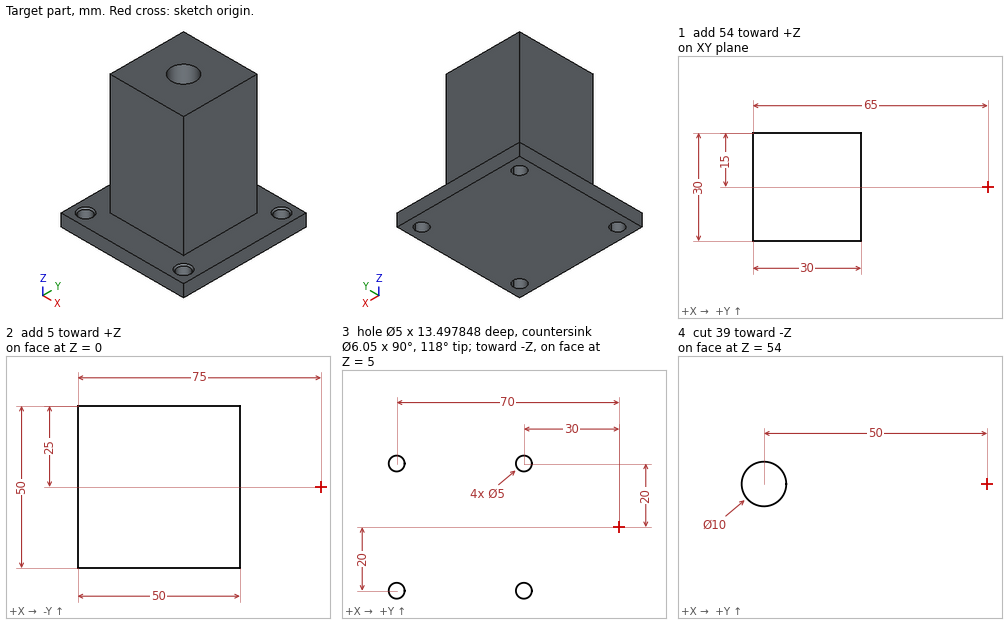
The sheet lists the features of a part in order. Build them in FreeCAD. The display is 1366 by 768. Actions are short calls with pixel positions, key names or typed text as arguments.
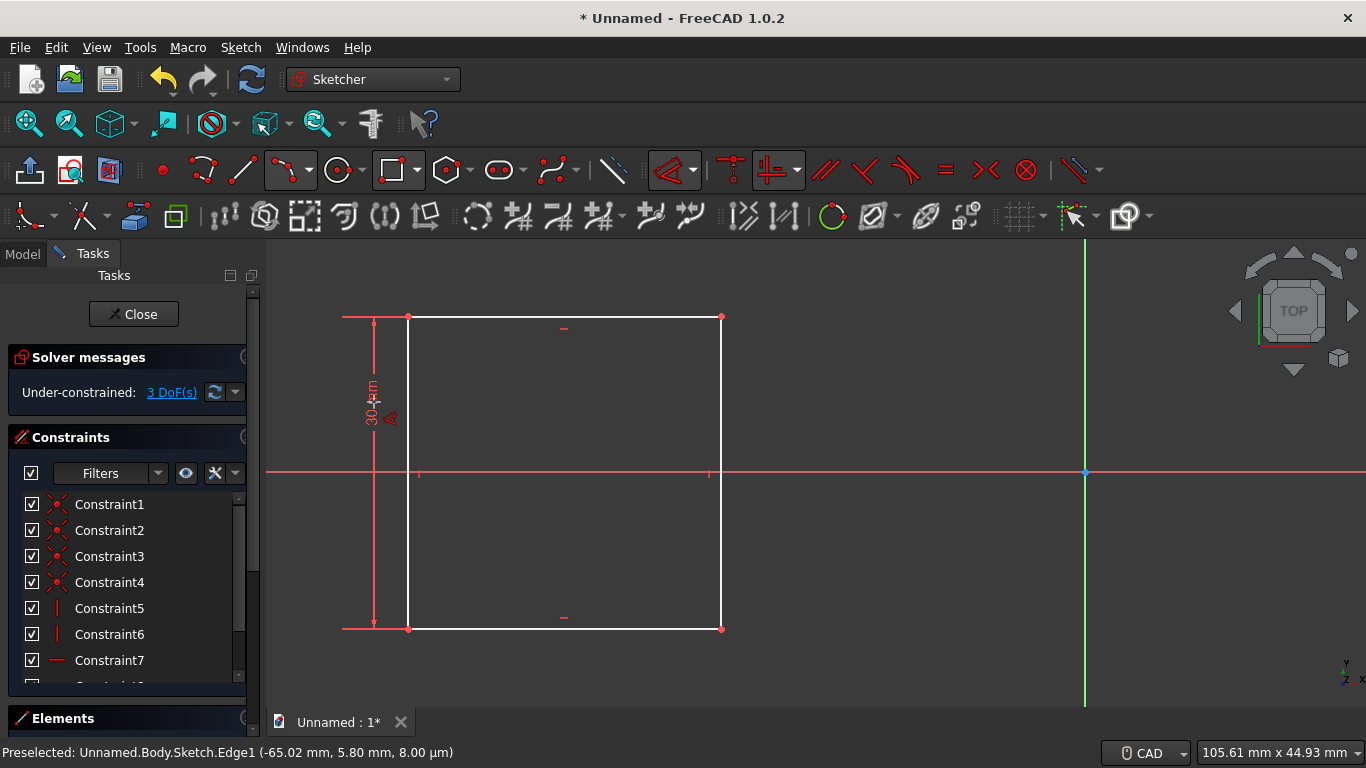
click(502, 629)
click(564, 663)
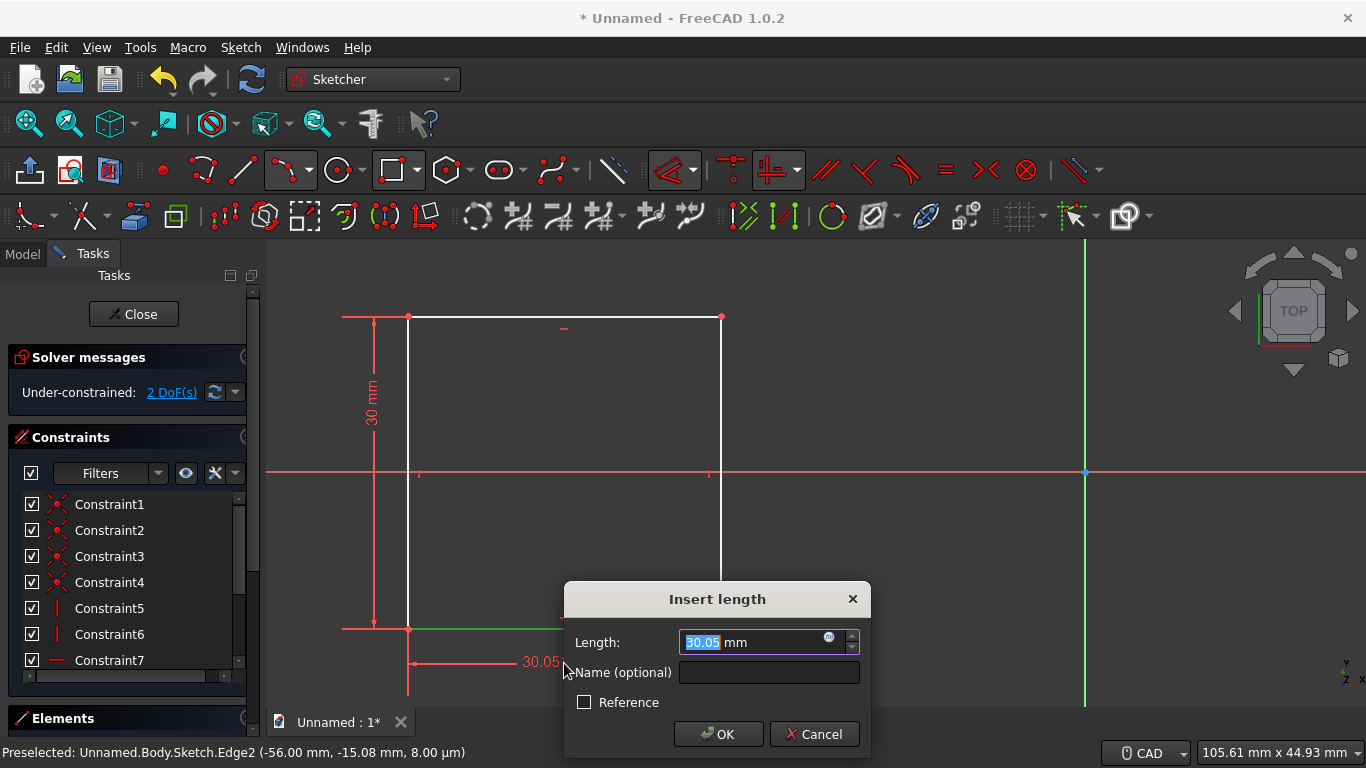
text(30)
key(Return)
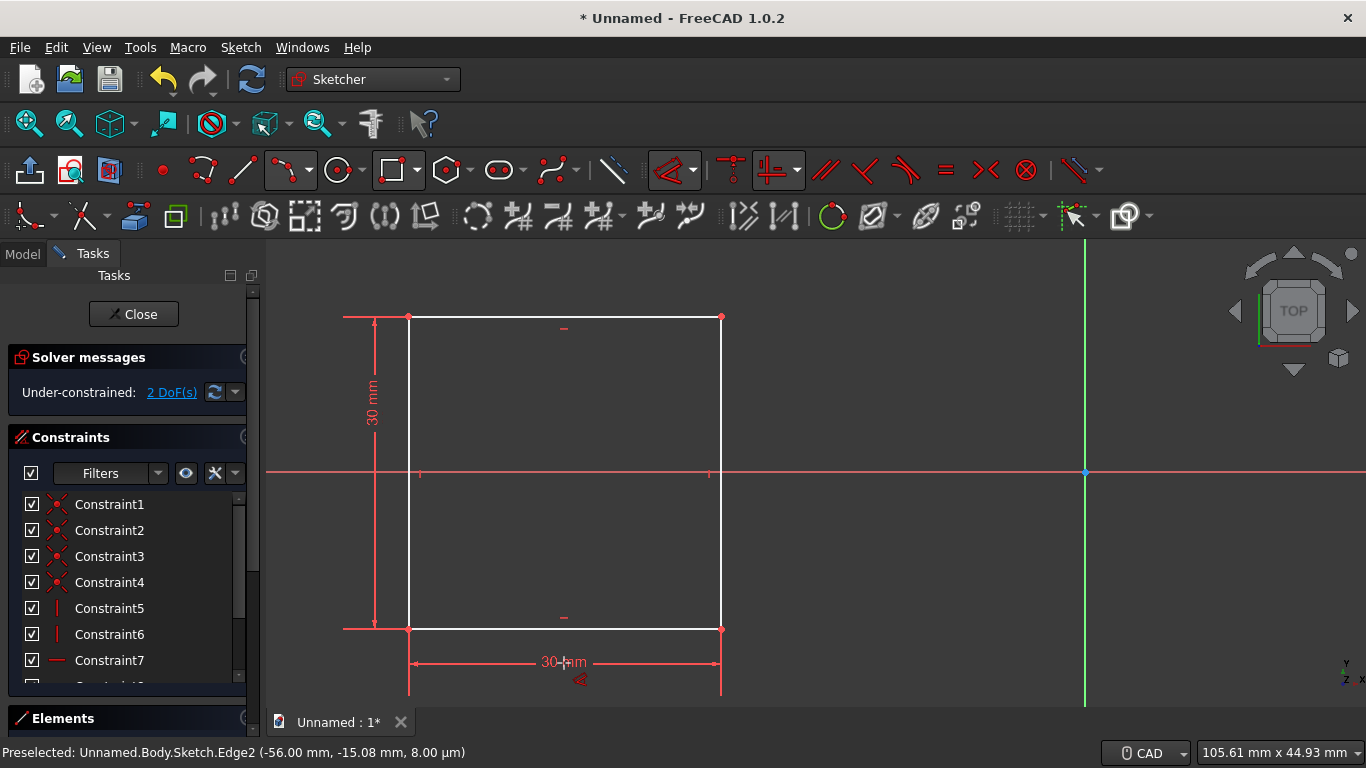
click(409, 317)
click(747, 283)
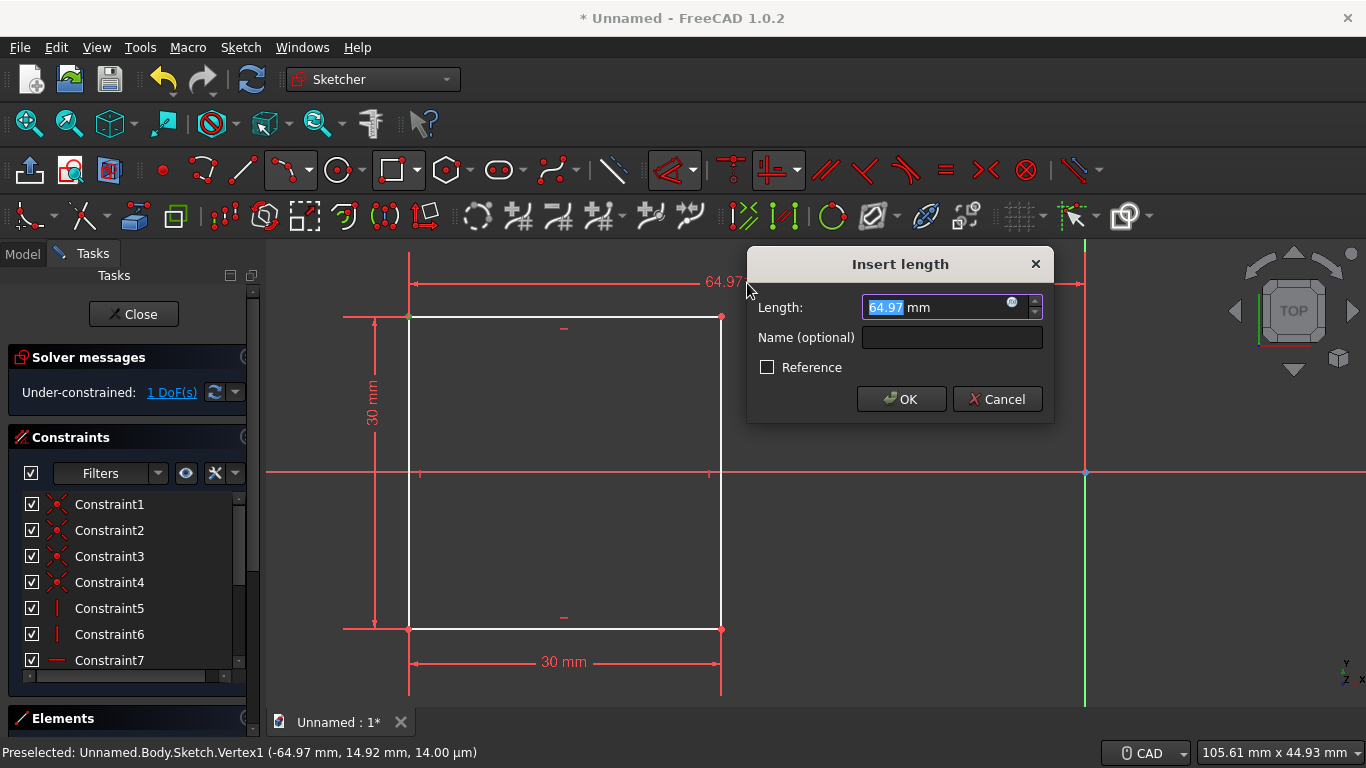
text(65)
key(Return)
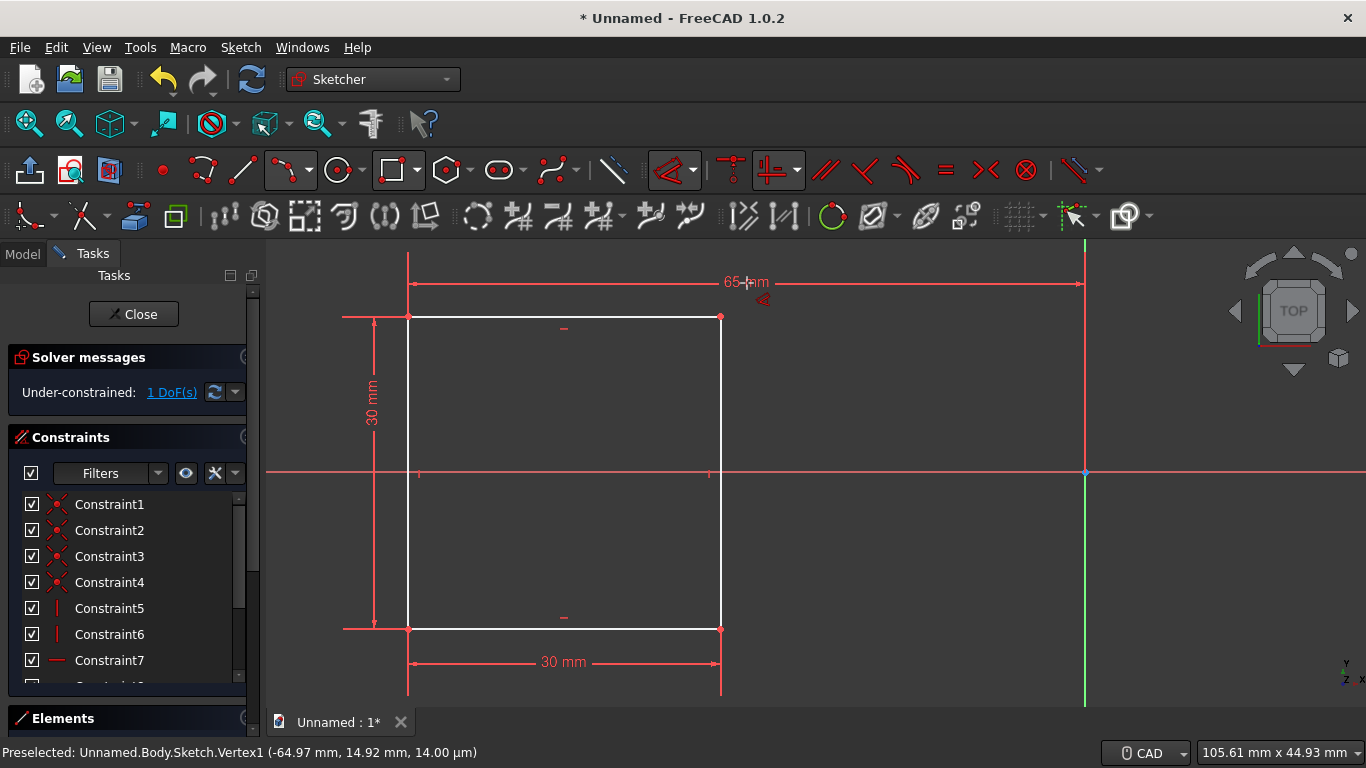
click(408, 317)
click(1119, 395)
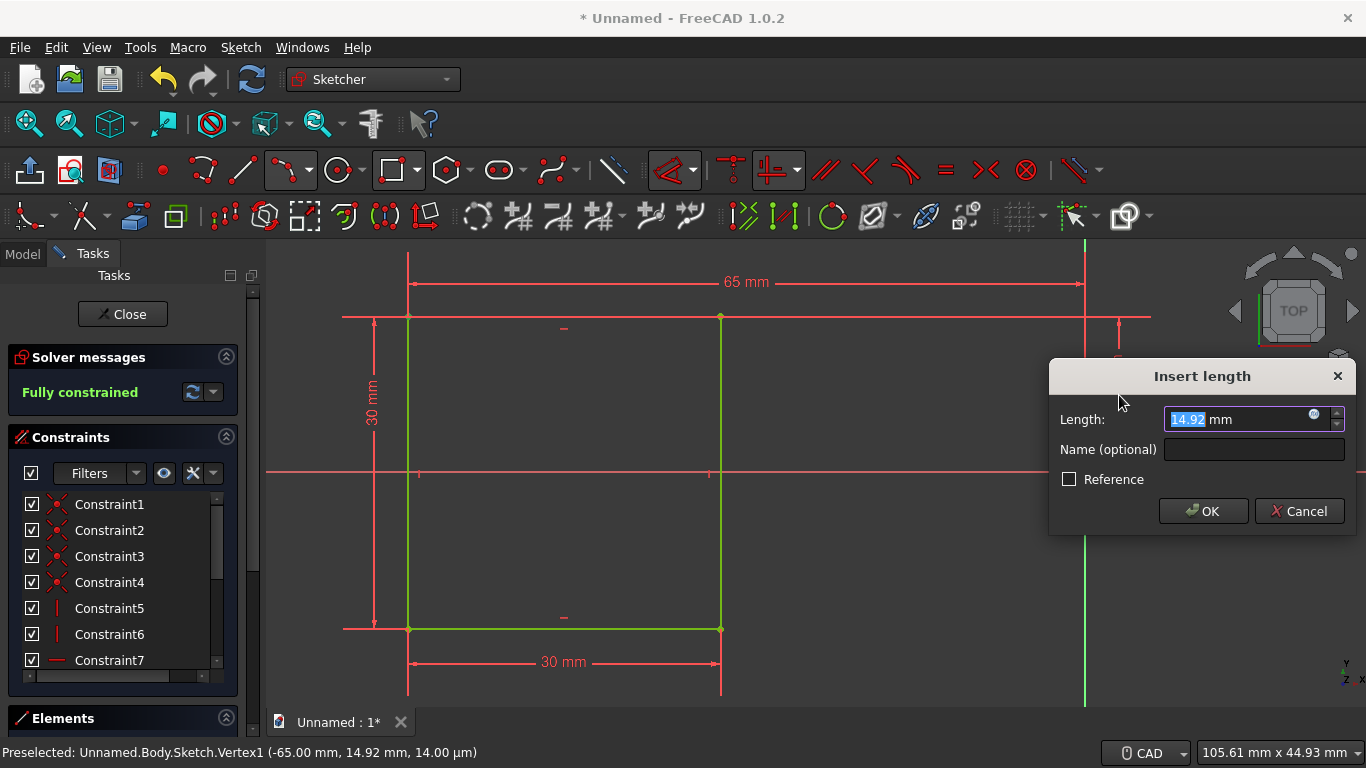
text(15)
key(Return)
key(Escape)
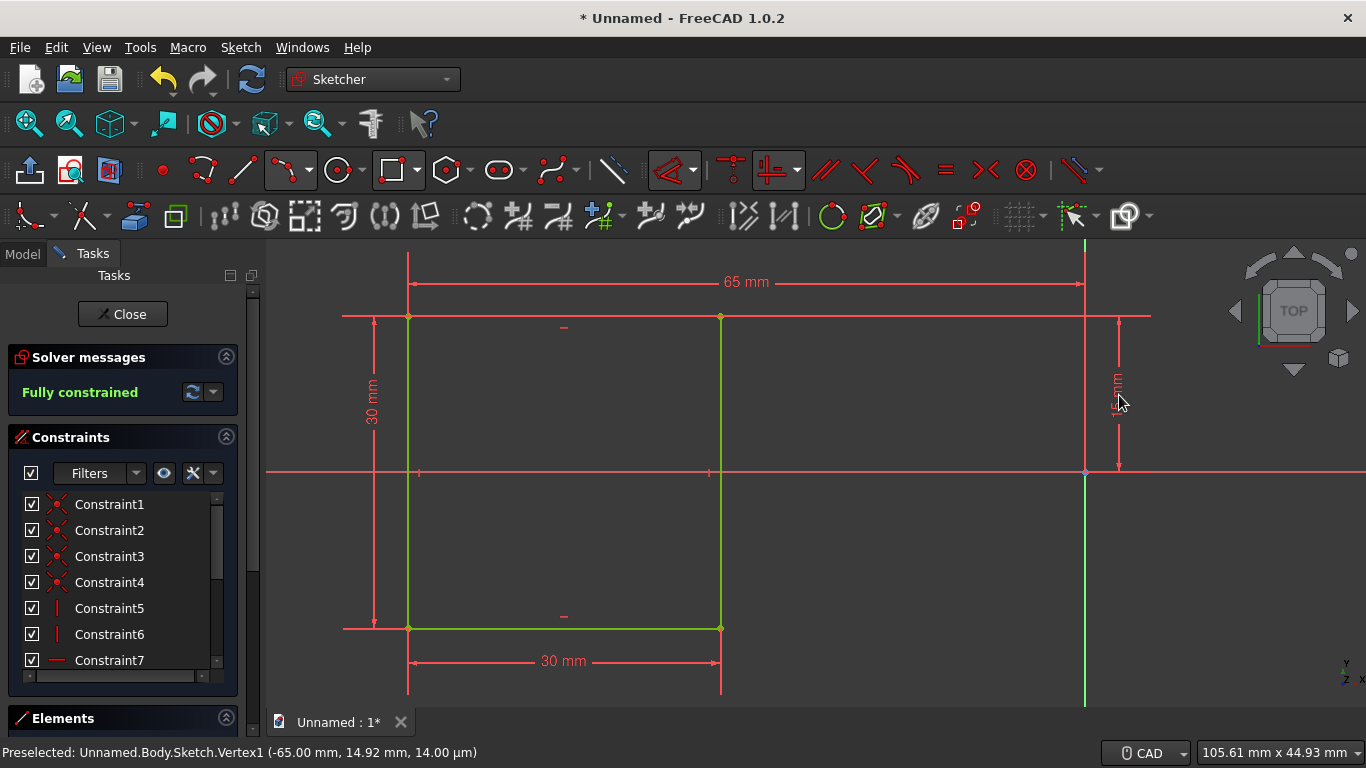
click(123, 314)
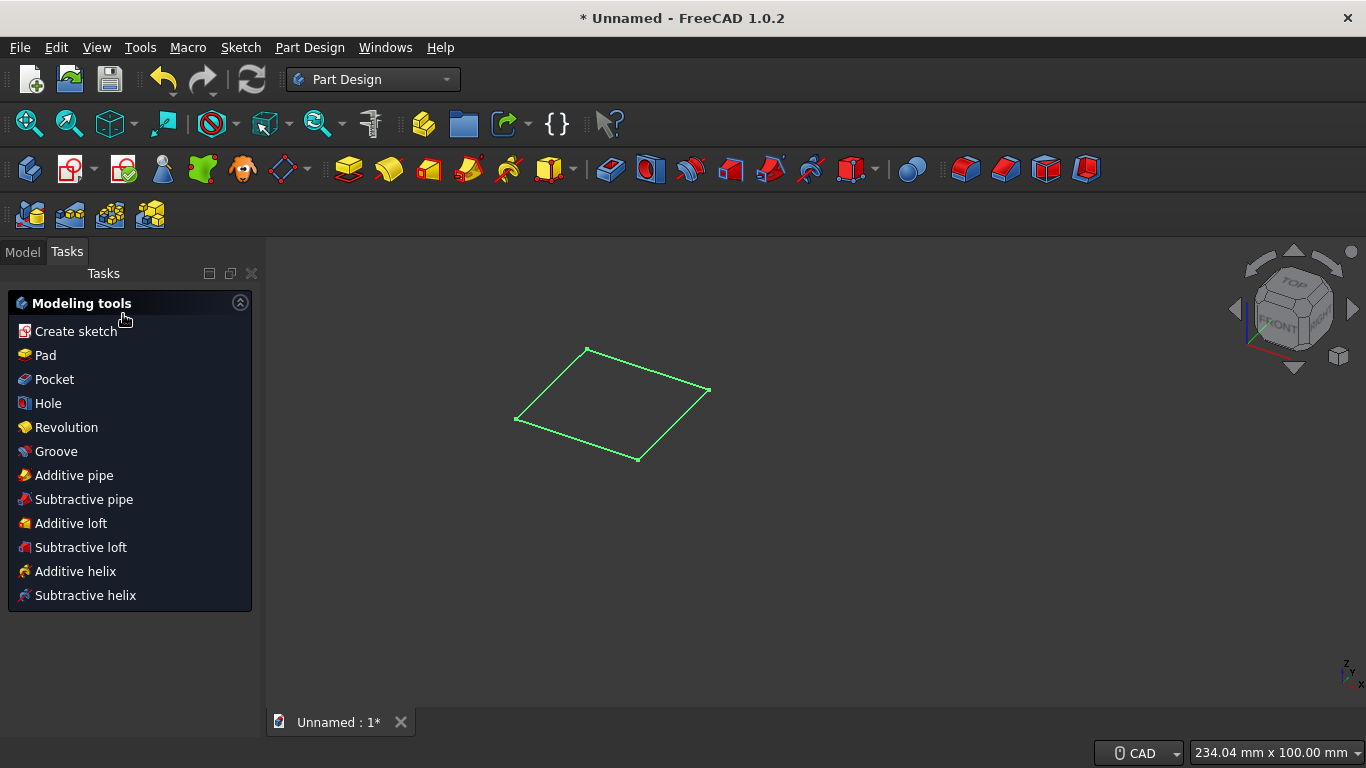
click(350, 170)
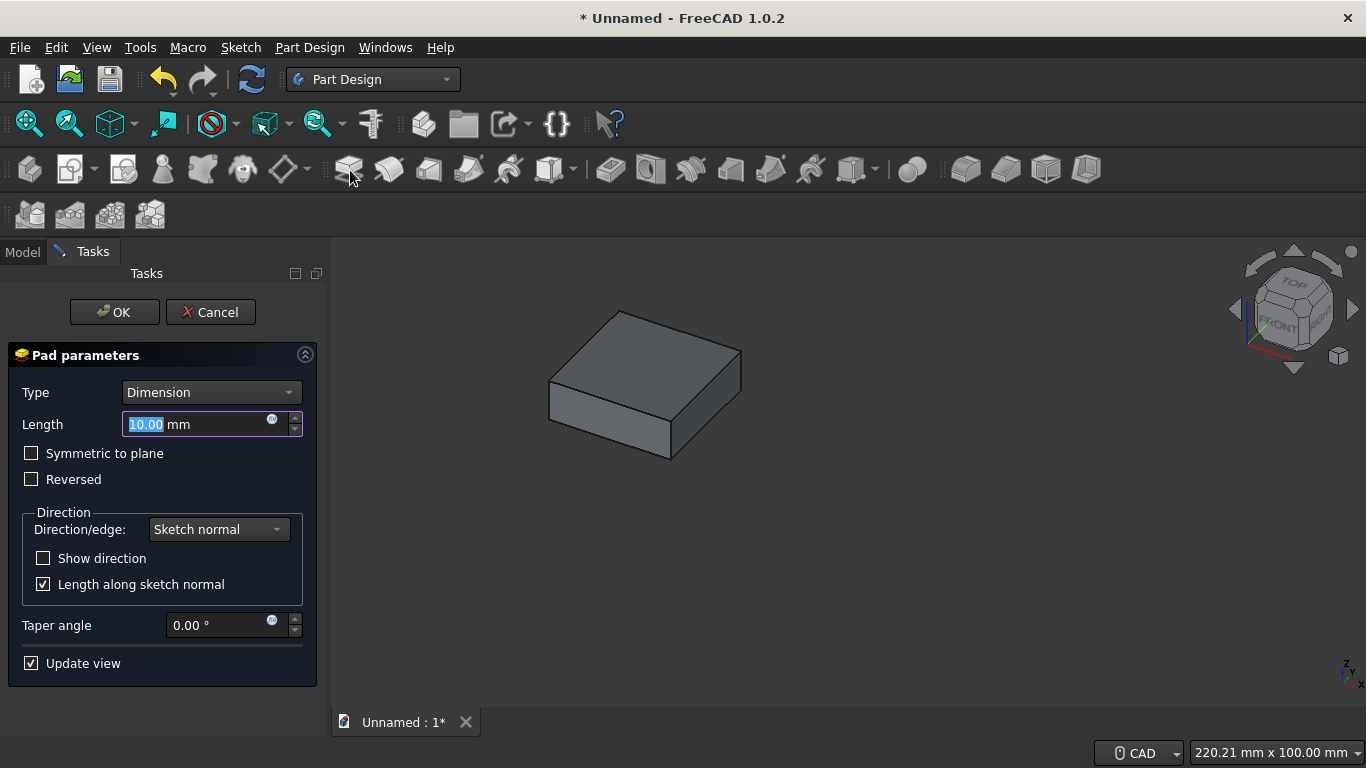
text(54)
key(Tab)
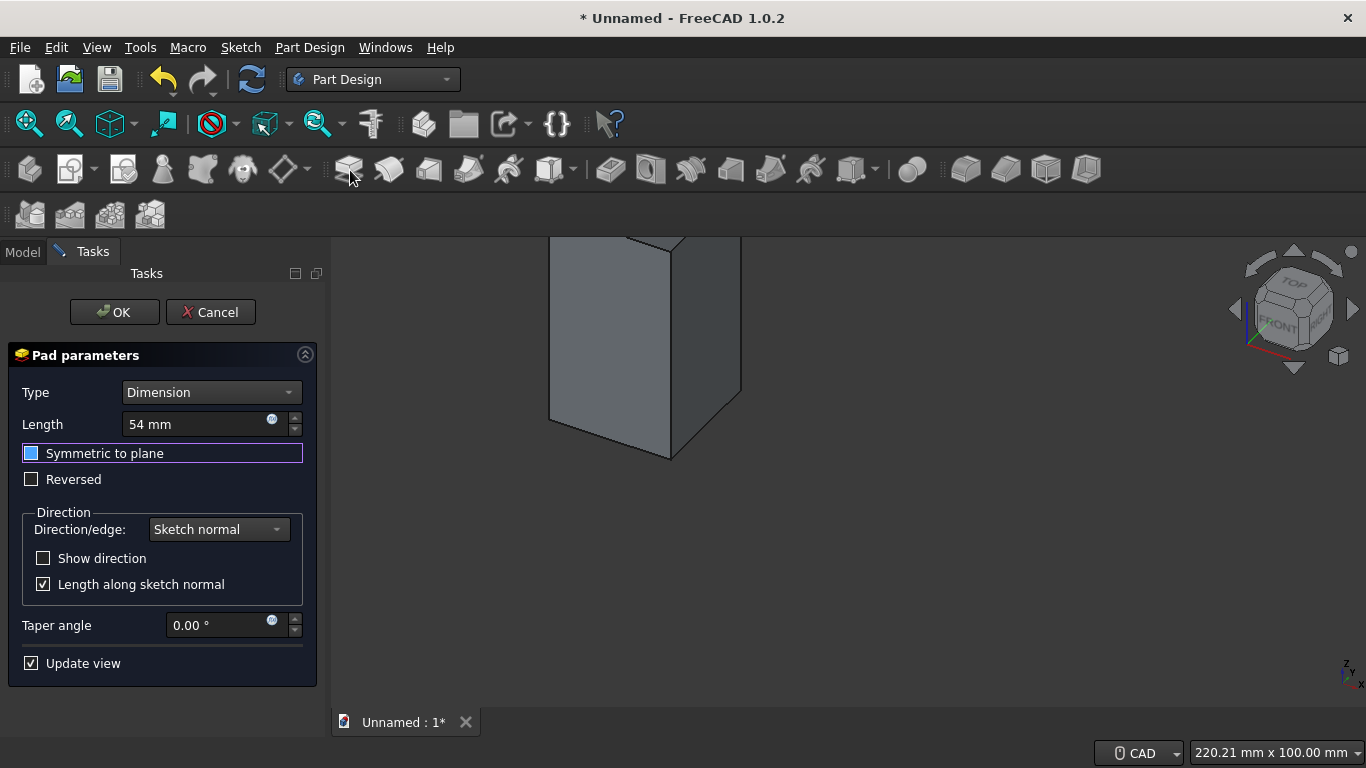
click(115, 312)